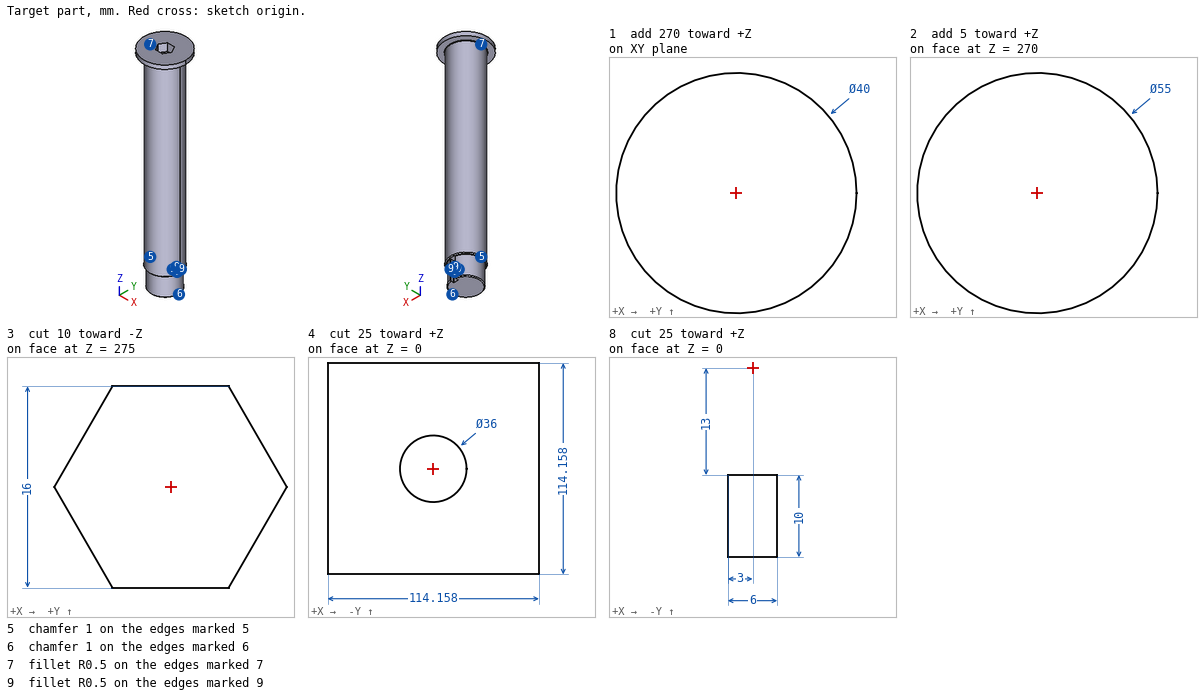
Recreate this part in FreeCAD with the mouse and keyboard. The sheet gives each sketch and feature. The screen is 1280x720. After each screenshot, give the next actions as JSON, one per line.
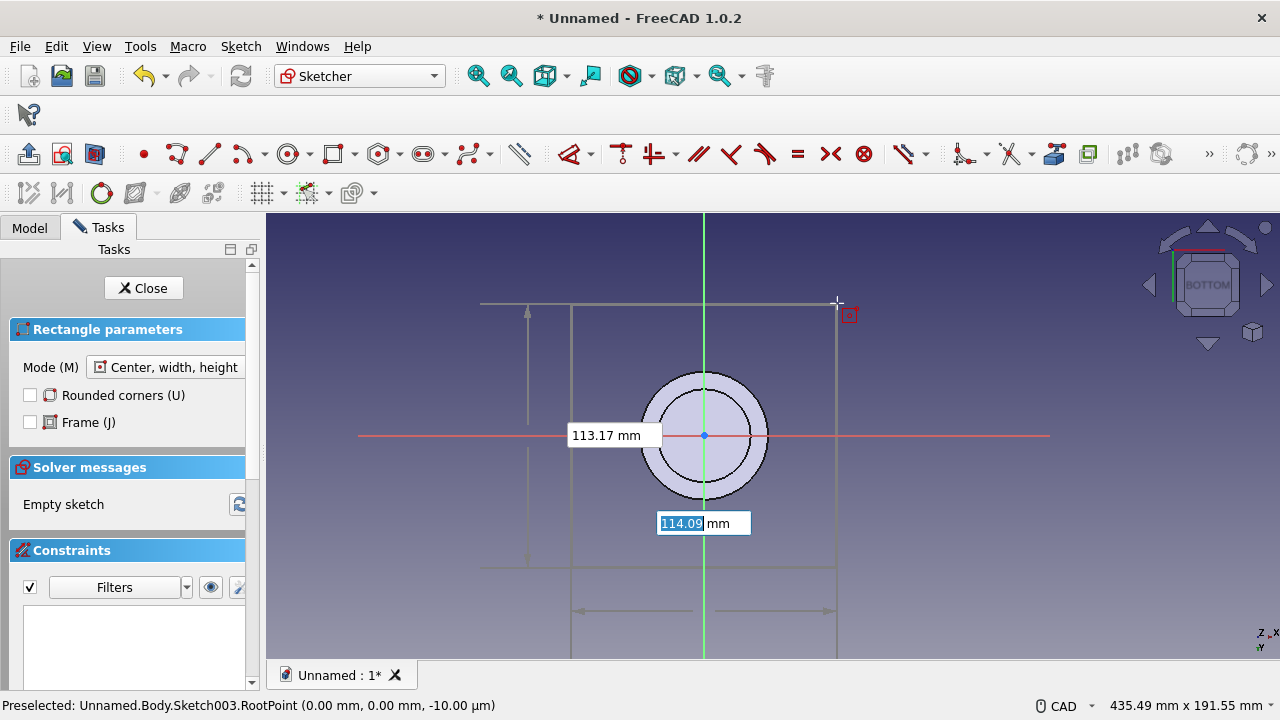
{"action": "type", "text": "114.158"}
{"action": "key", "text": "Tab"}
{"action": "type", "text": "114.158"}
{"action": "key", "text": "Return"}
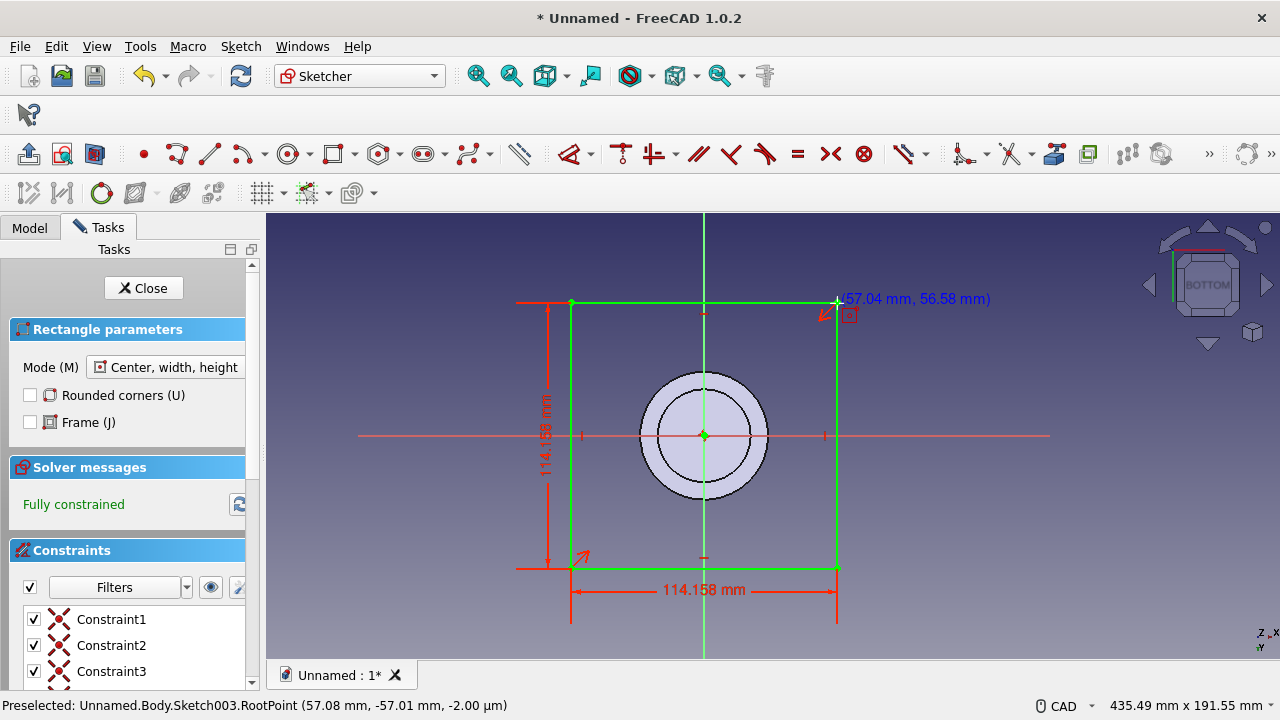
{"action": "left_click", "coordinate": [288, 154]}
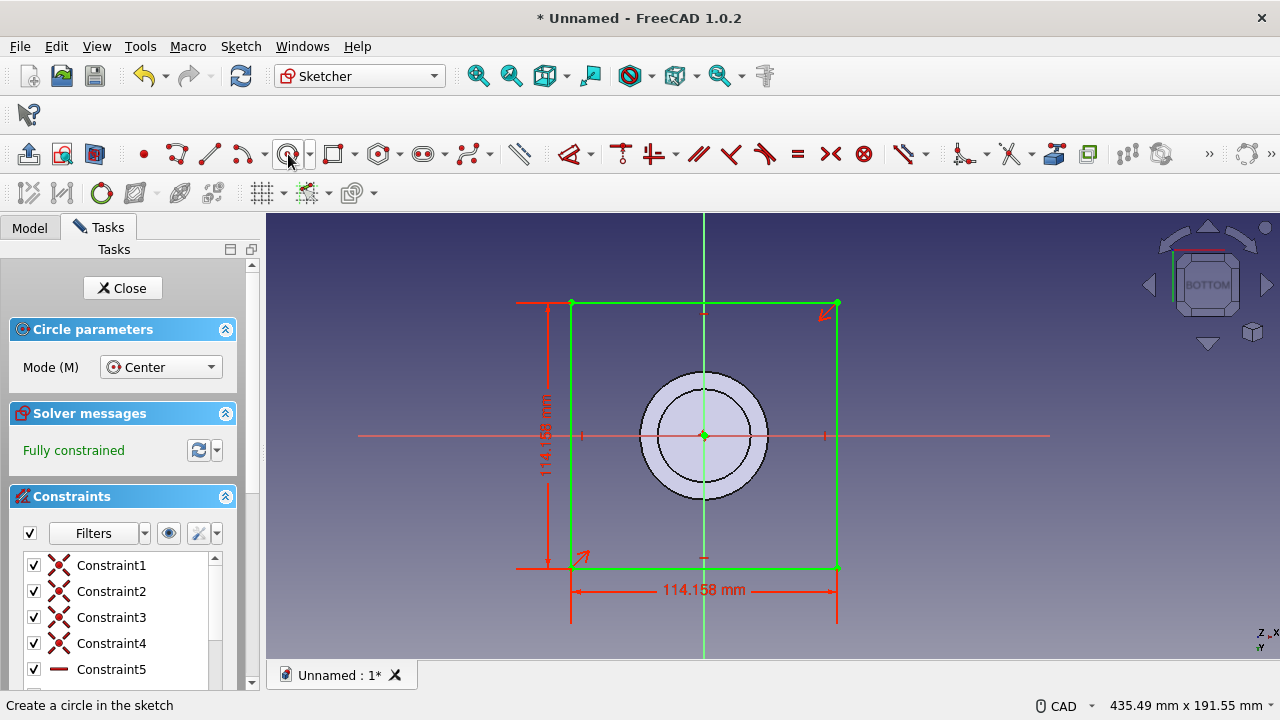
{"action": "left_click", "coordinate": [704, 436]}
{"action": "mouse_move", "coordinate": [734, 406]}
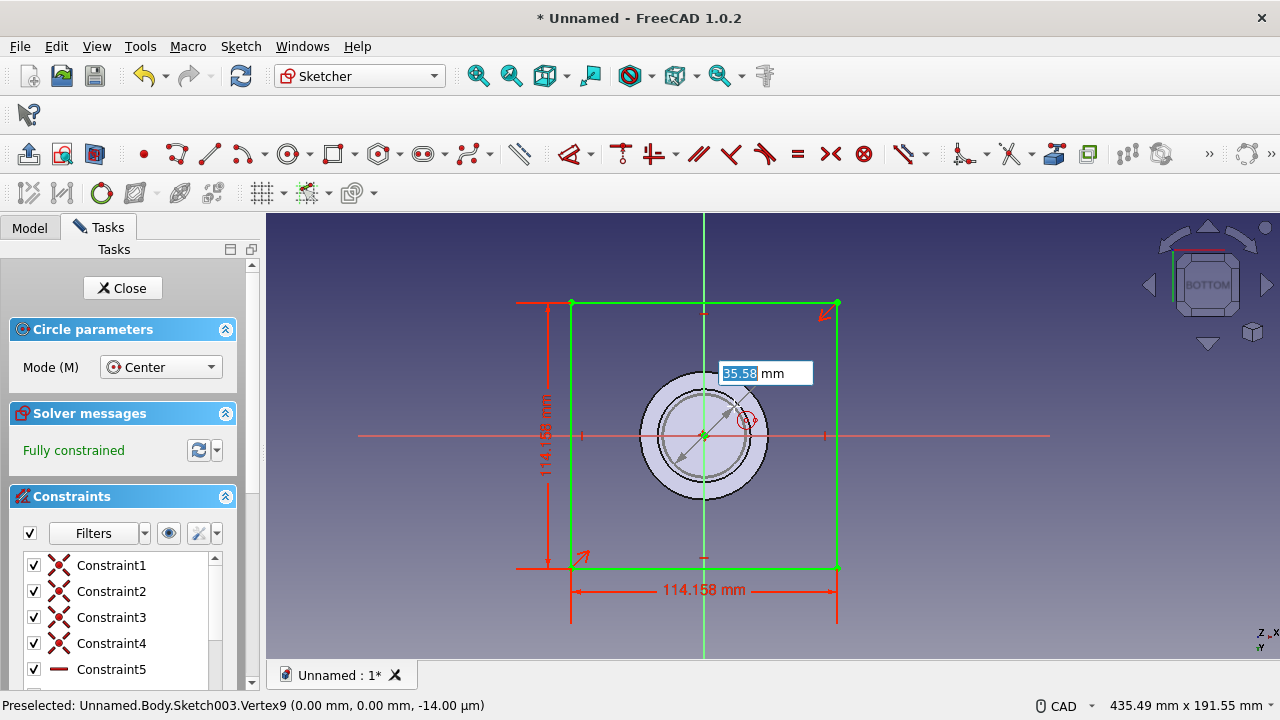
{"action": "type", "text": "36"}
{"action": "key", "text": "Return"}
{"action": "key", "text": "Escape"}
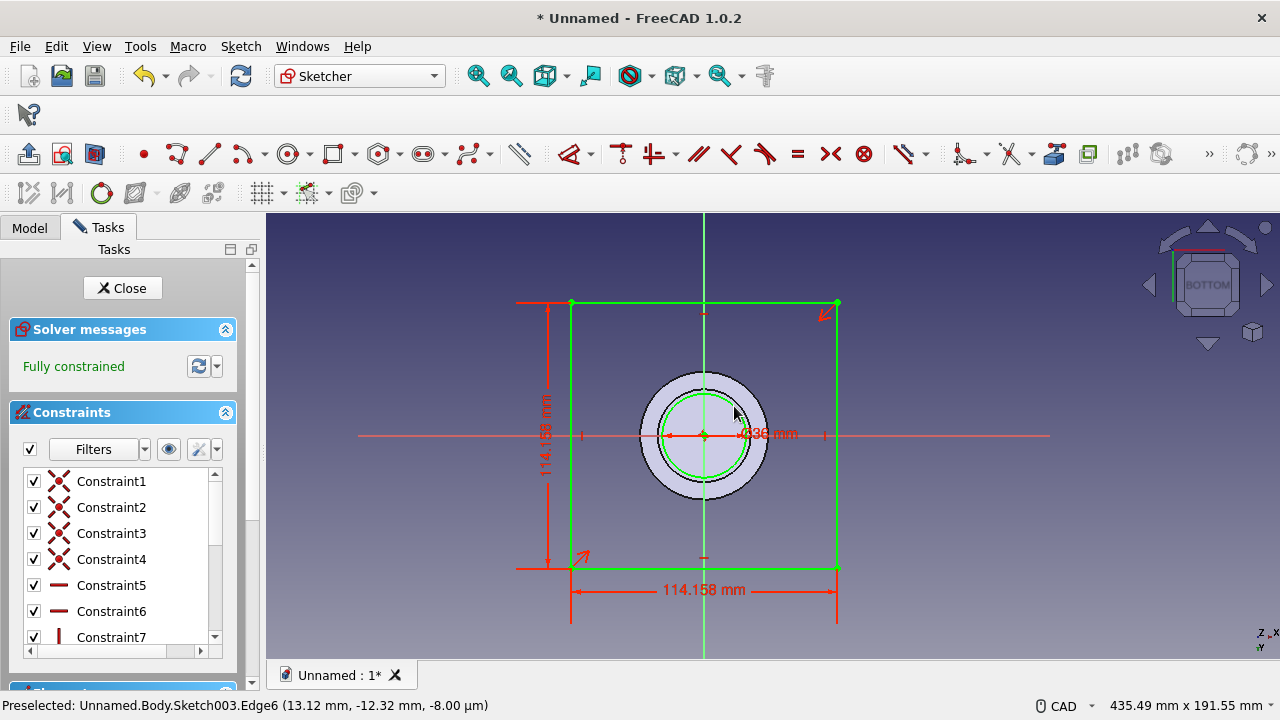
{"action": "left_click", "coordinate": [123, 288]}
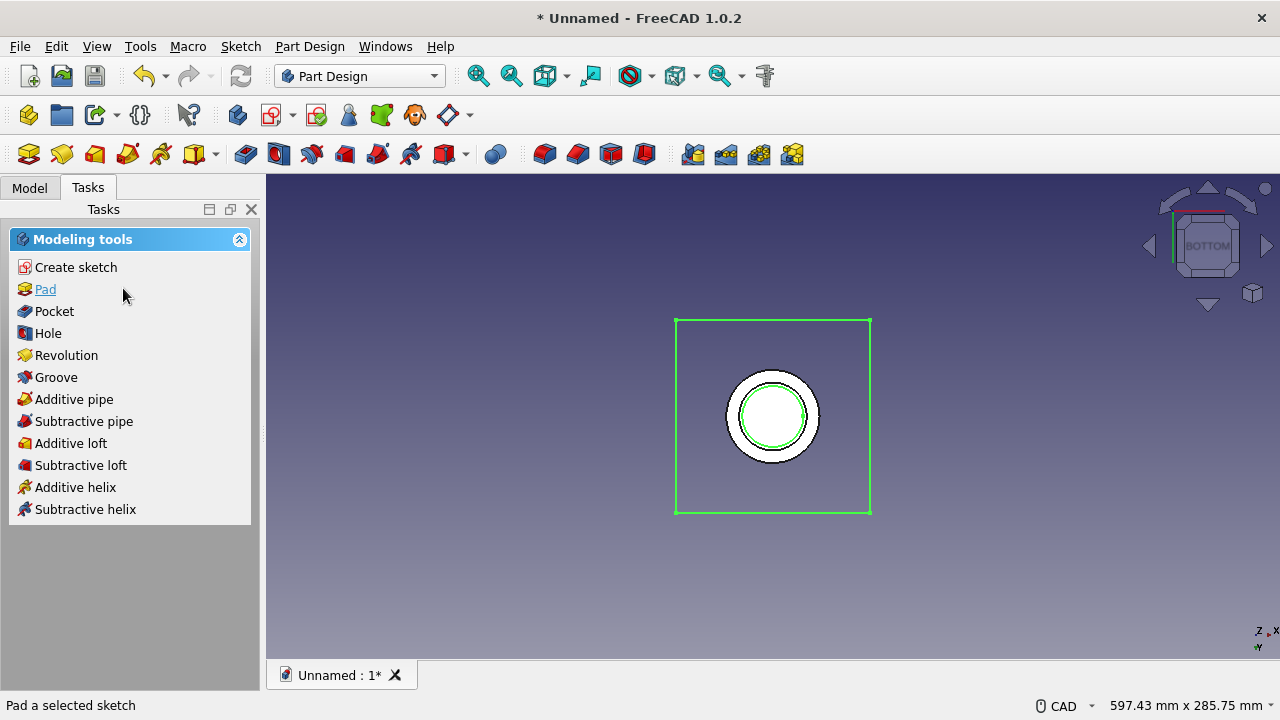
{"action": "left_click", "coordinate": [246, 154]}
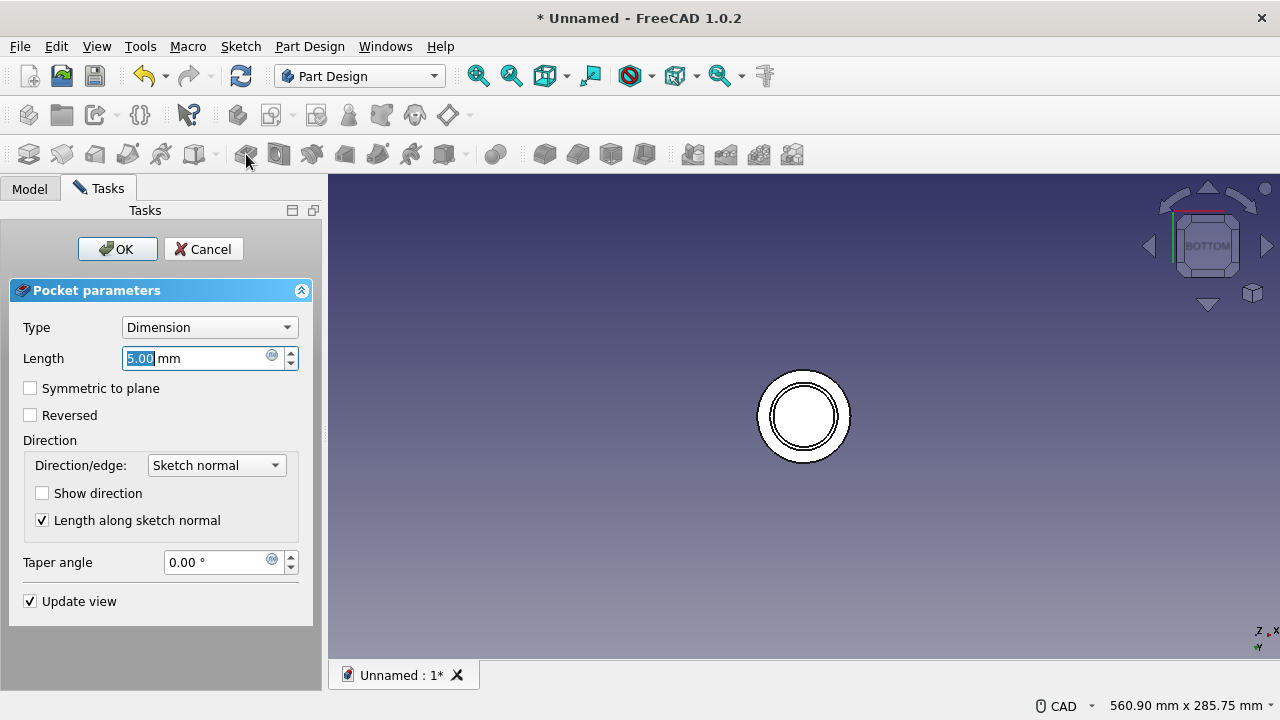
{"action": "type", "text": "25"}
{"action": "key", "text": "Tab"}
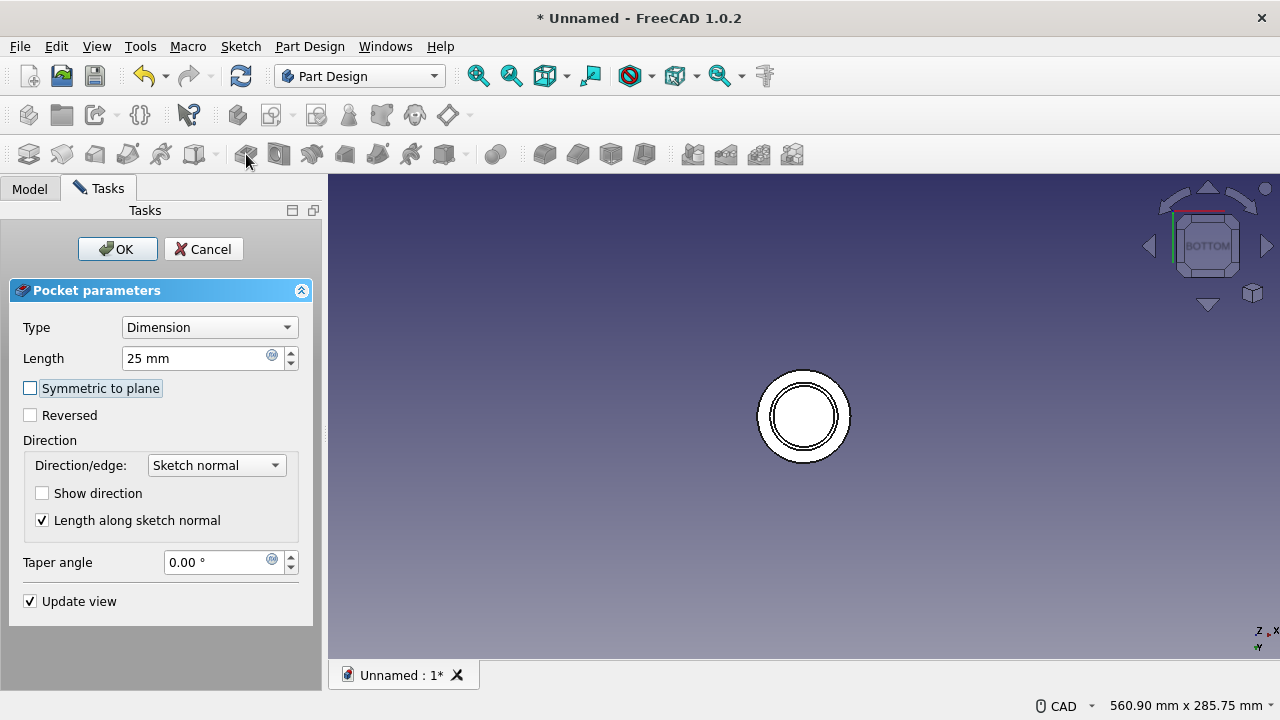
{"action": "left_click", "coordinate": [118, 249]}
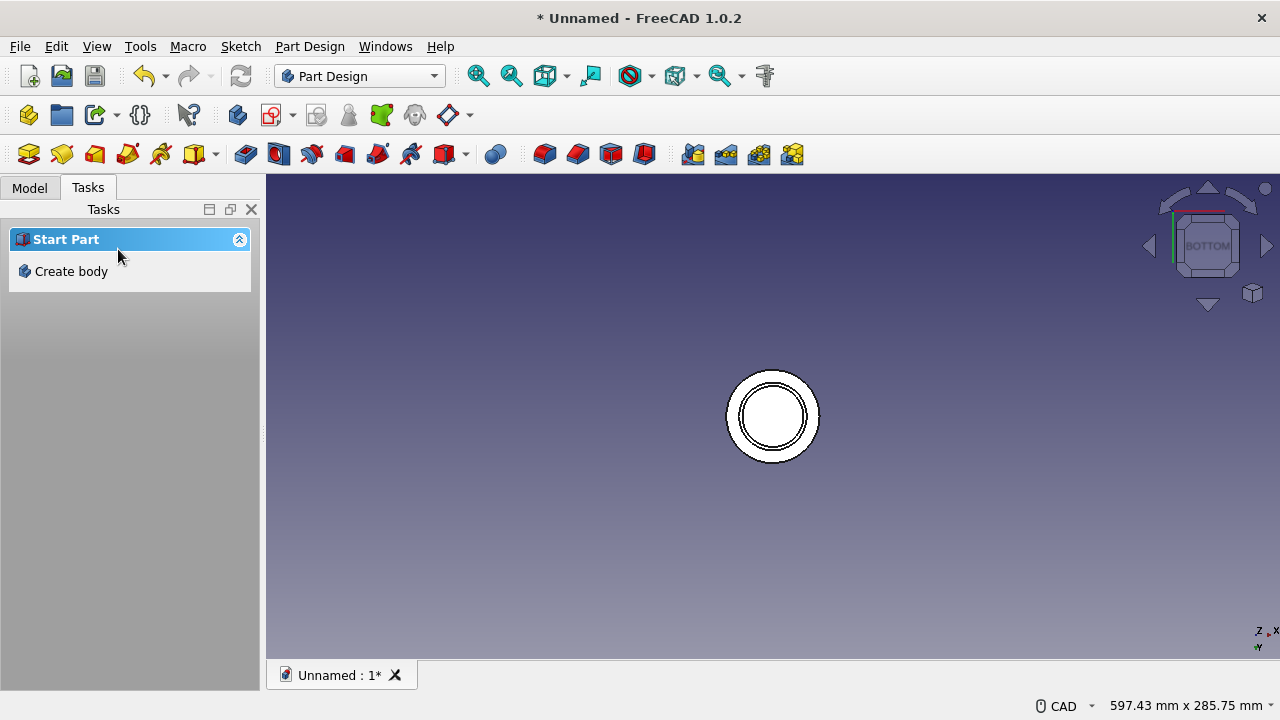
{"action": "left_click", "coordinate": [479, 76]}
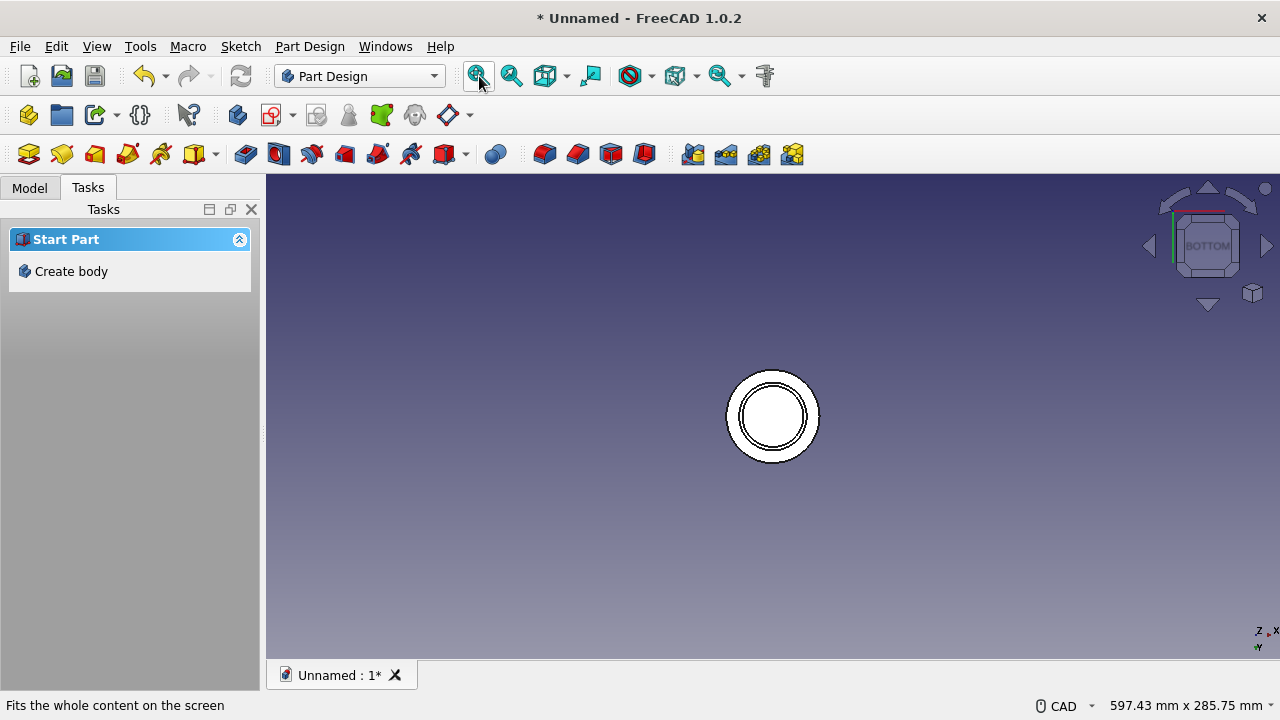
{"action": "key", "text": "0"}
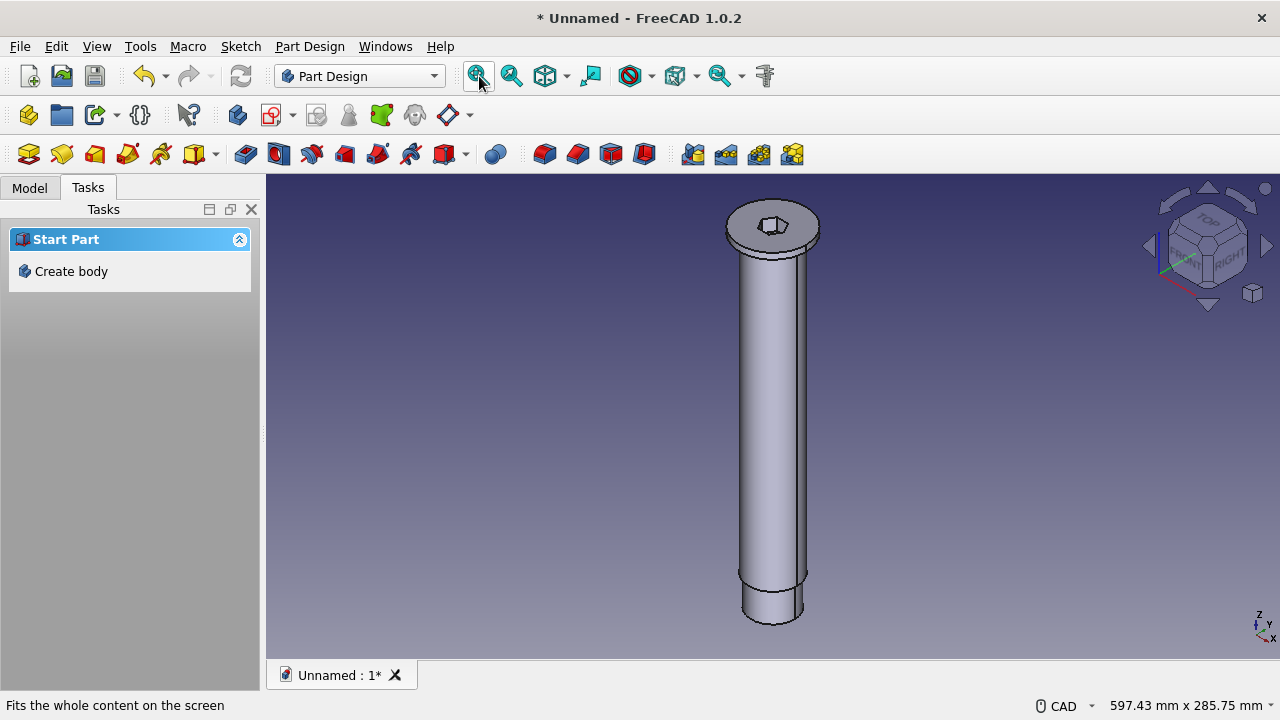
{"action": "key", "text": "2"}